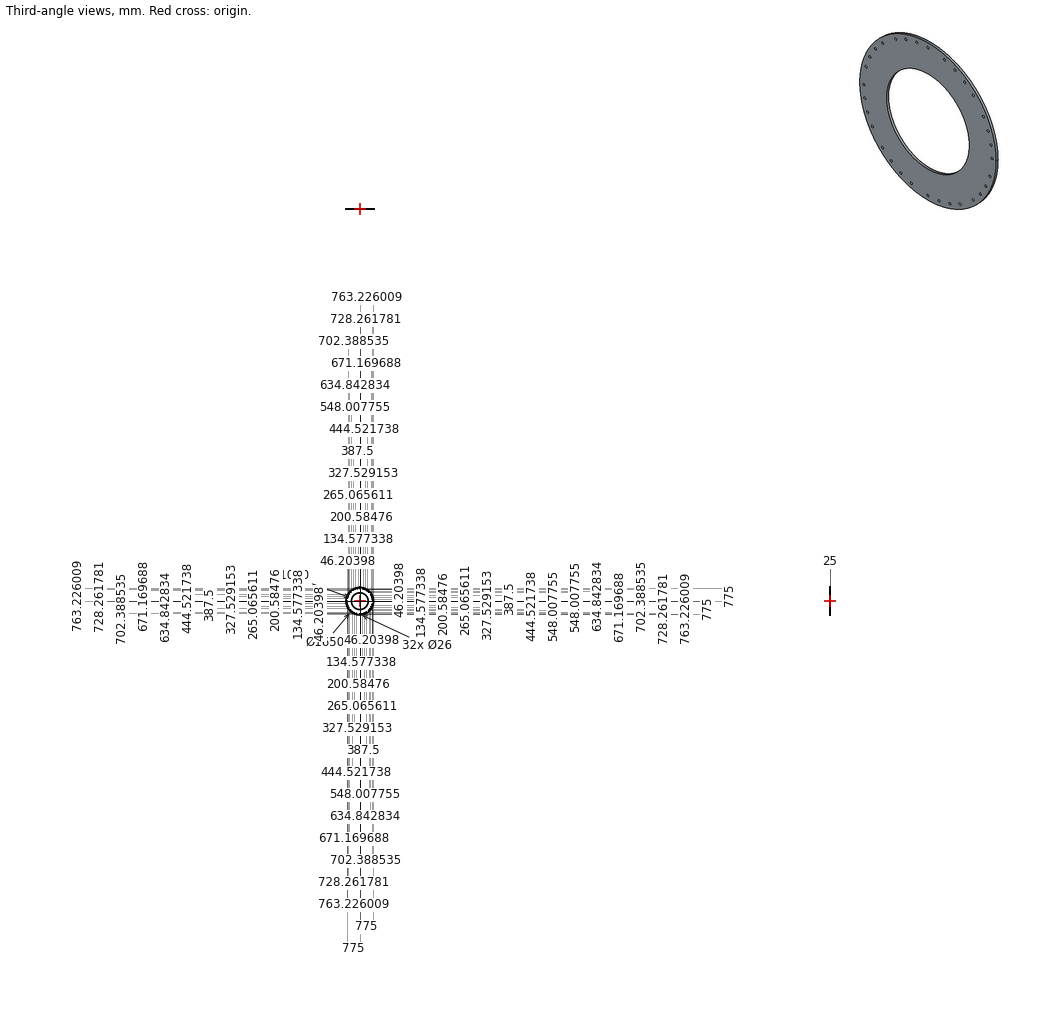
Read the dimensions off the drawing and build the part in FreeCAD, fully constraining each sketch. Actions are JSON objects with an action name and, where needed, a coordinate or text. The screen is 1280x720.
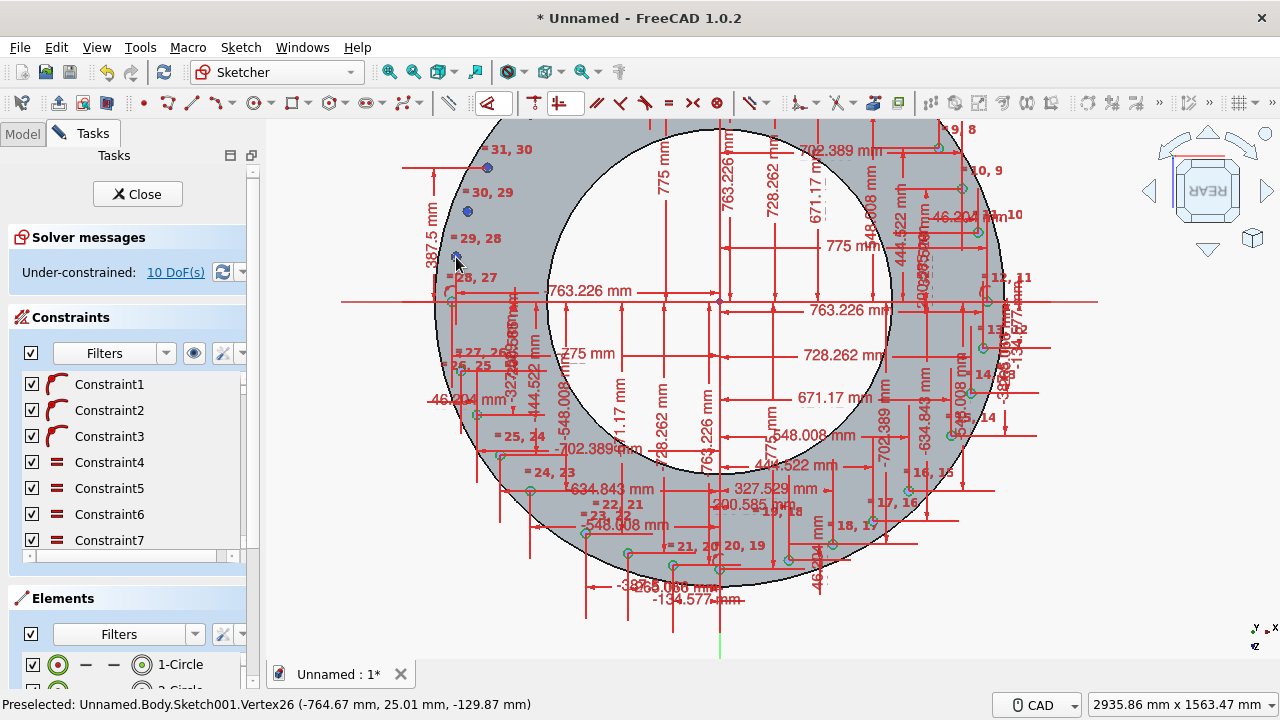
{"action": "left_click", "coordinate": [456, 257]}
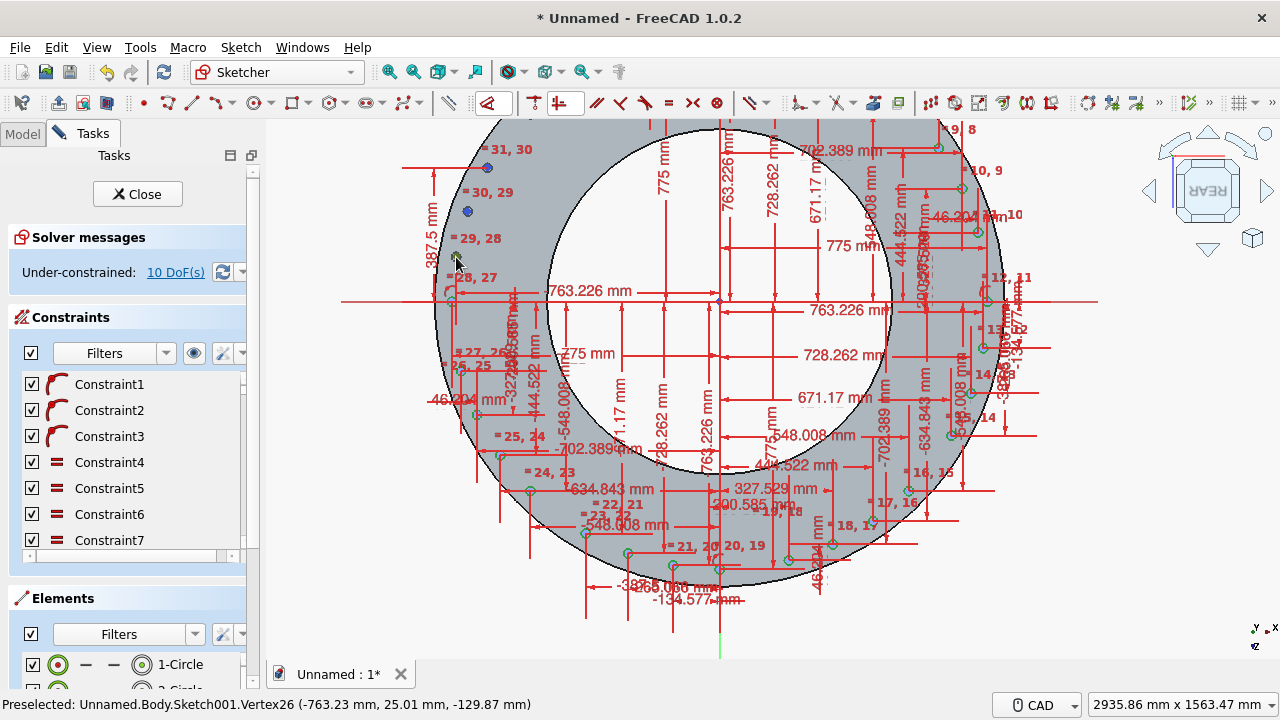
{"action": "key", "text": "i"}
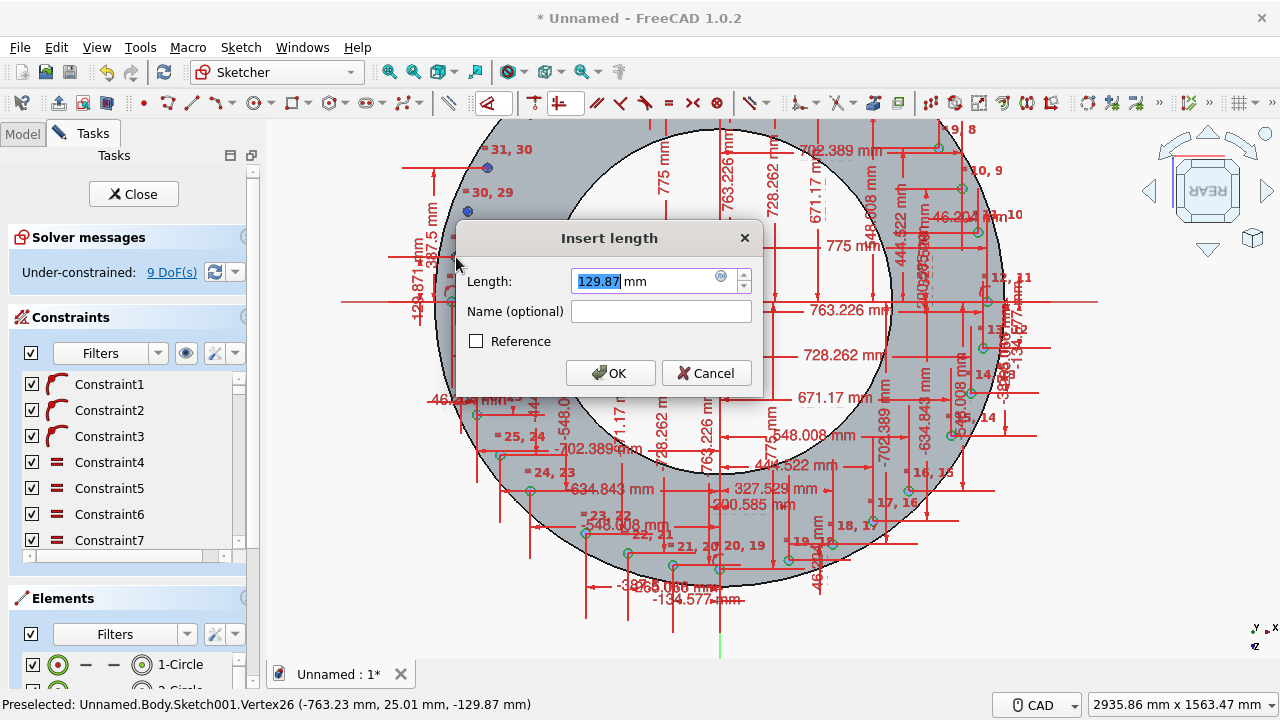
{"action": "type", "text": "134.577338"}
{"action": "key", "text": "Return"}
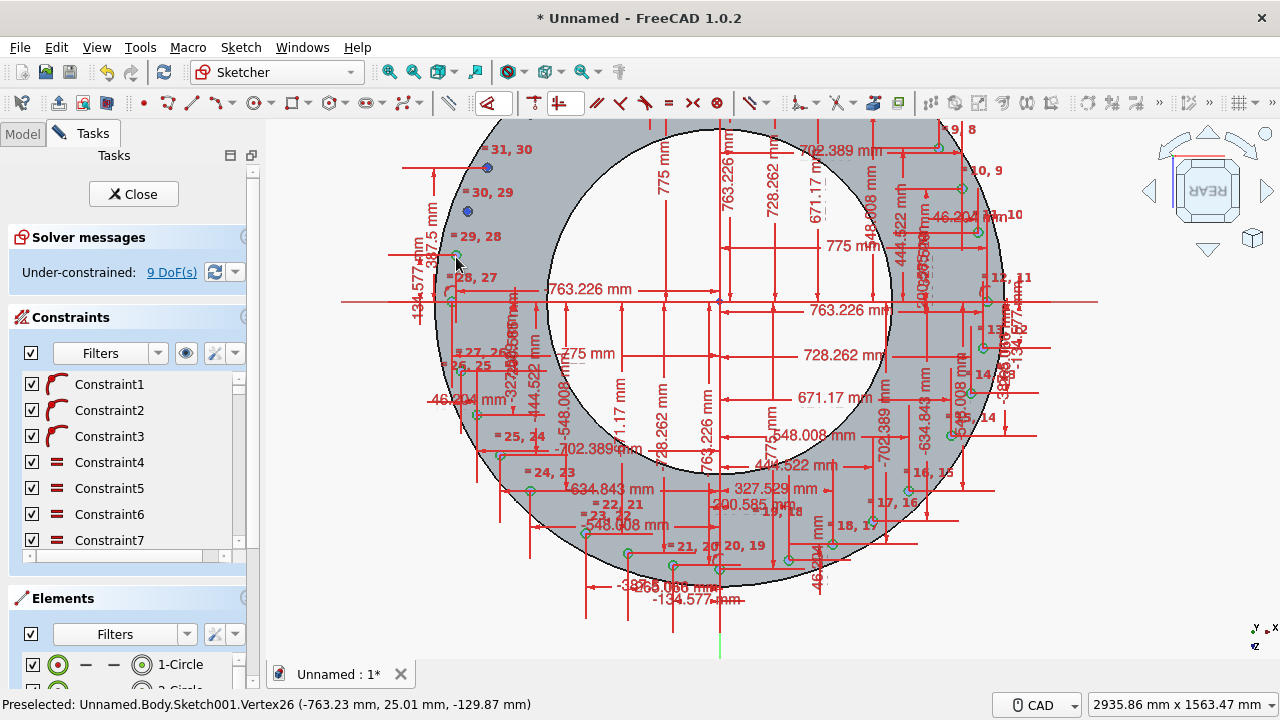
{"action": "left_click", "coordinate": [468, 211]}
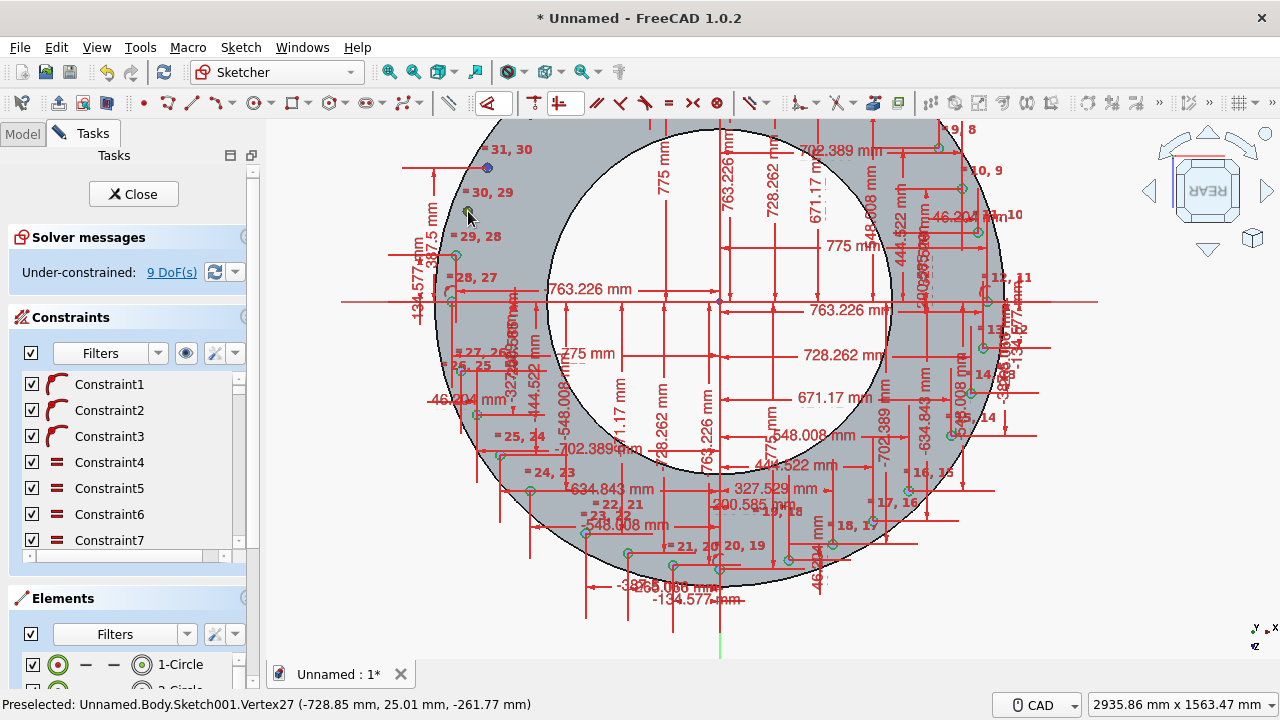
{"action": "left_click", "coordinate": [506, 104]}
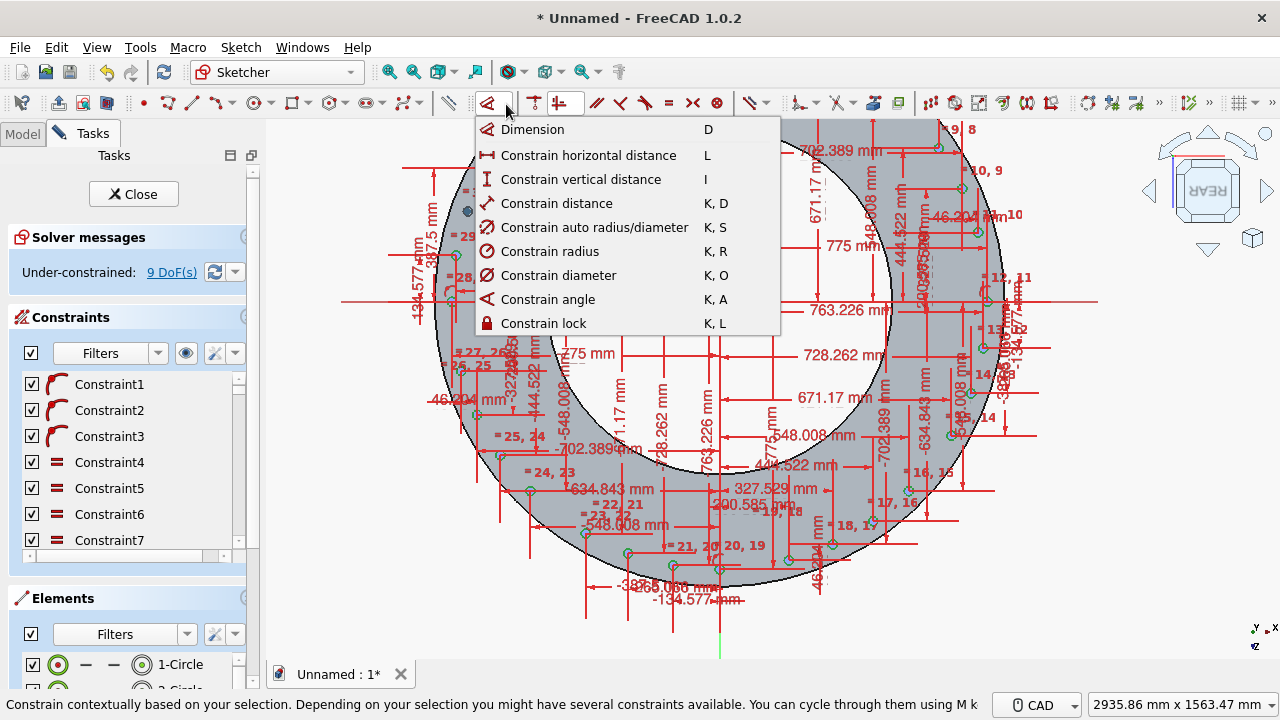
{"action": "left_click", "coordinate": [628, 155]}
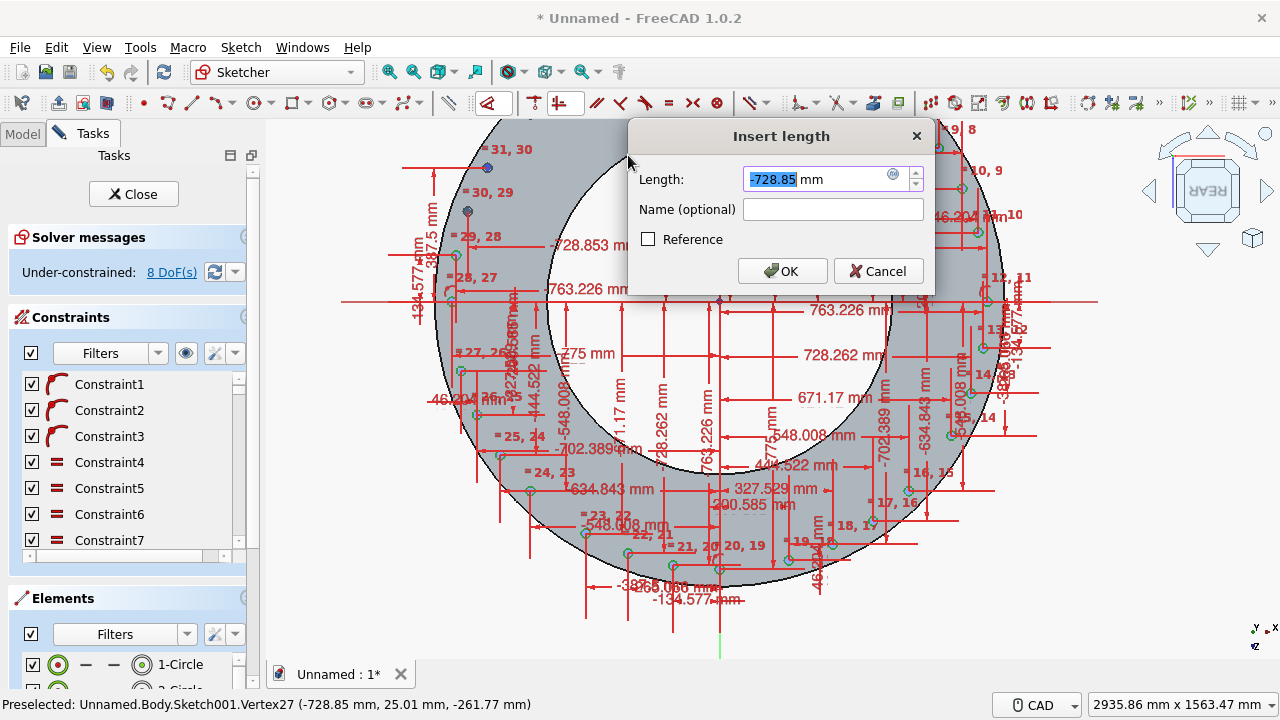
{"action": "type", "text": "-728.261781"}
{"action": "key", "text": "Return"}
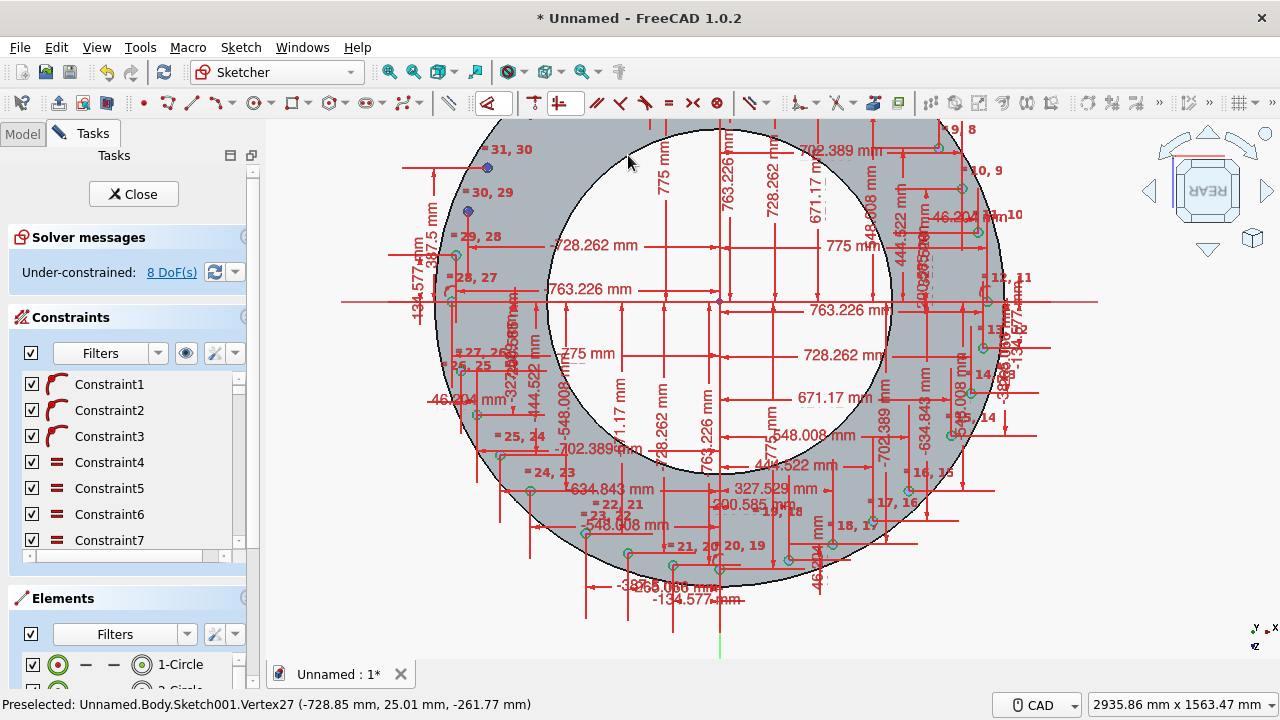
{"action": "left_click", "coordinate": [468, 211]}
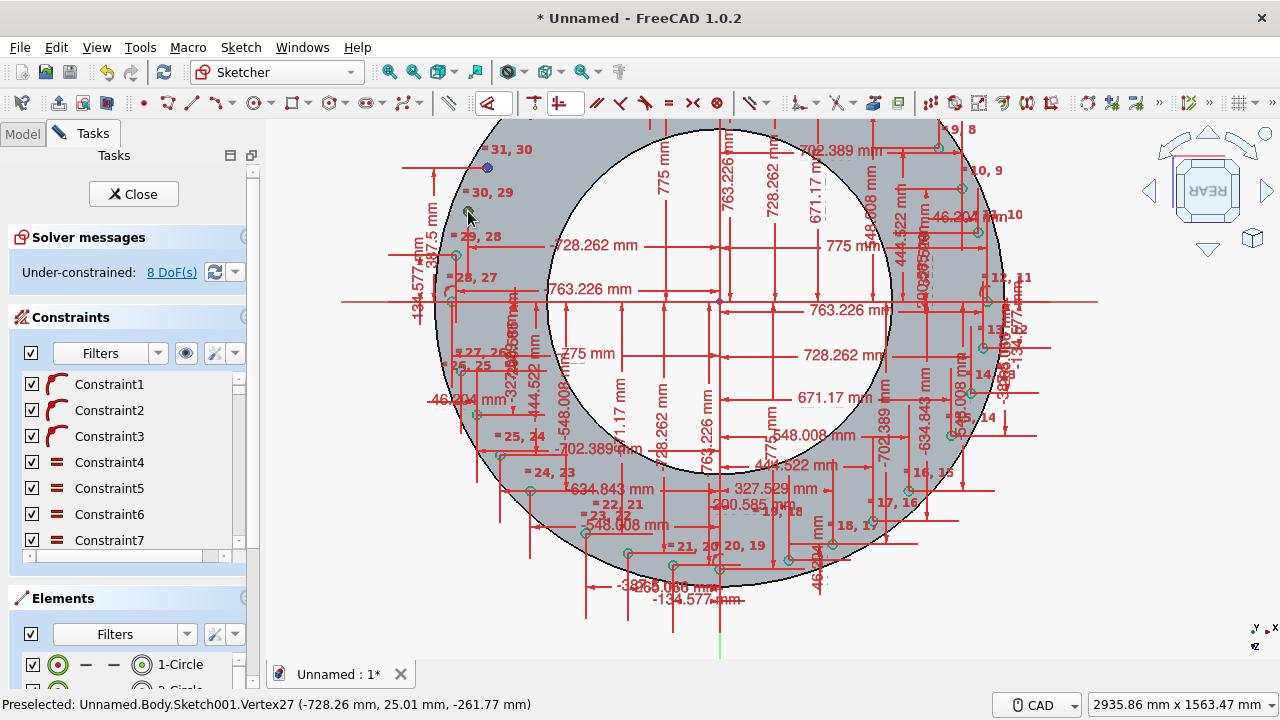
{"action": "key", "text": "i"}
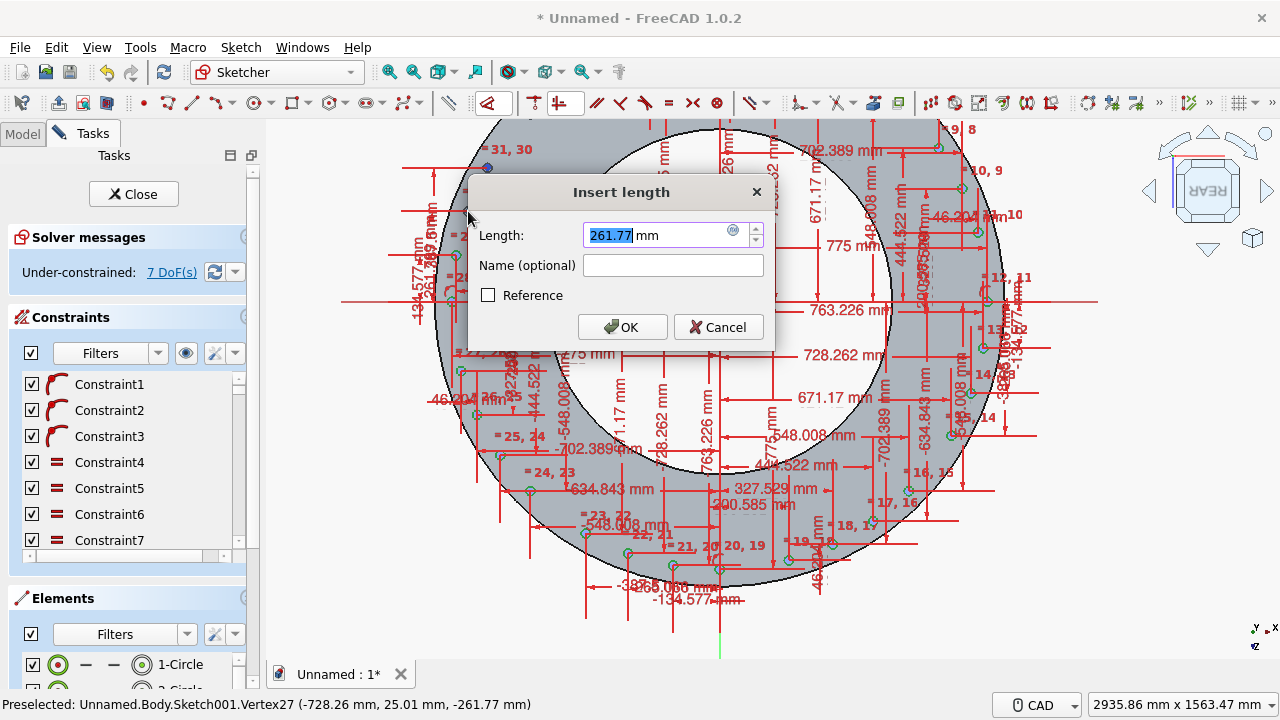
{"action": "type", "text": "265.065611"}
{"action": "key", "text": "Return"}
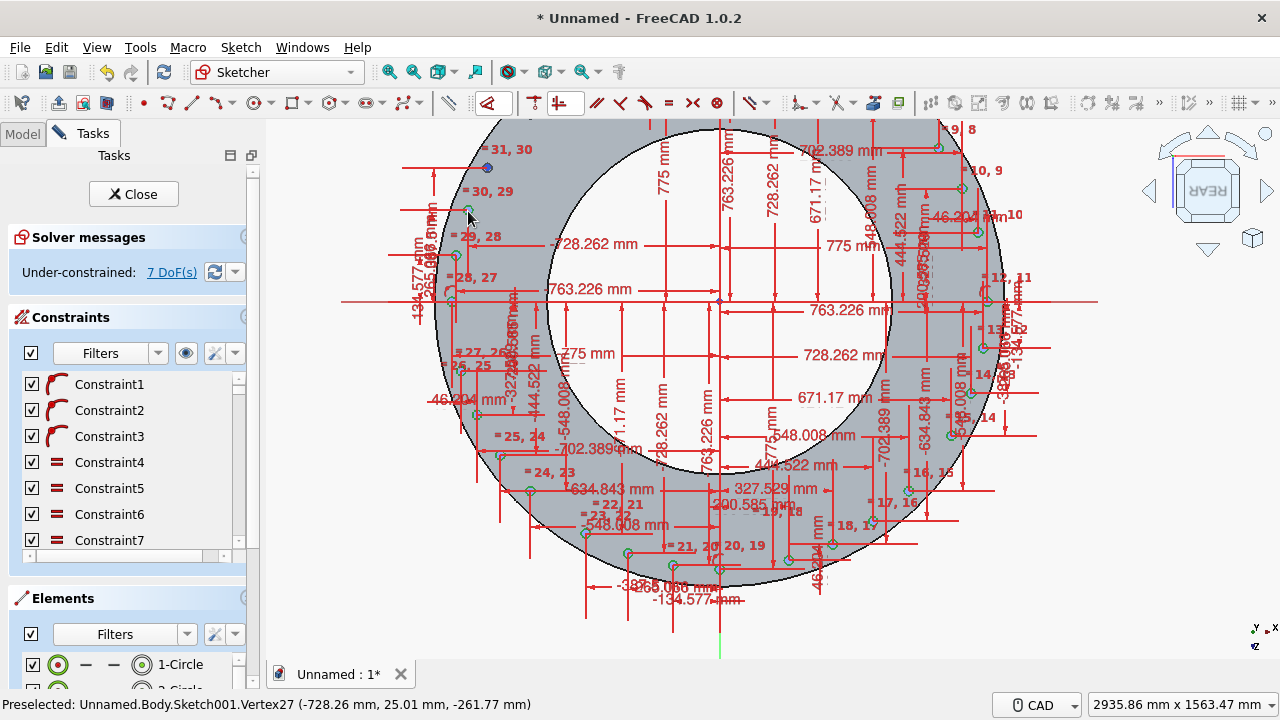
{"action": "left_click", "coordinate": [487, 168]}